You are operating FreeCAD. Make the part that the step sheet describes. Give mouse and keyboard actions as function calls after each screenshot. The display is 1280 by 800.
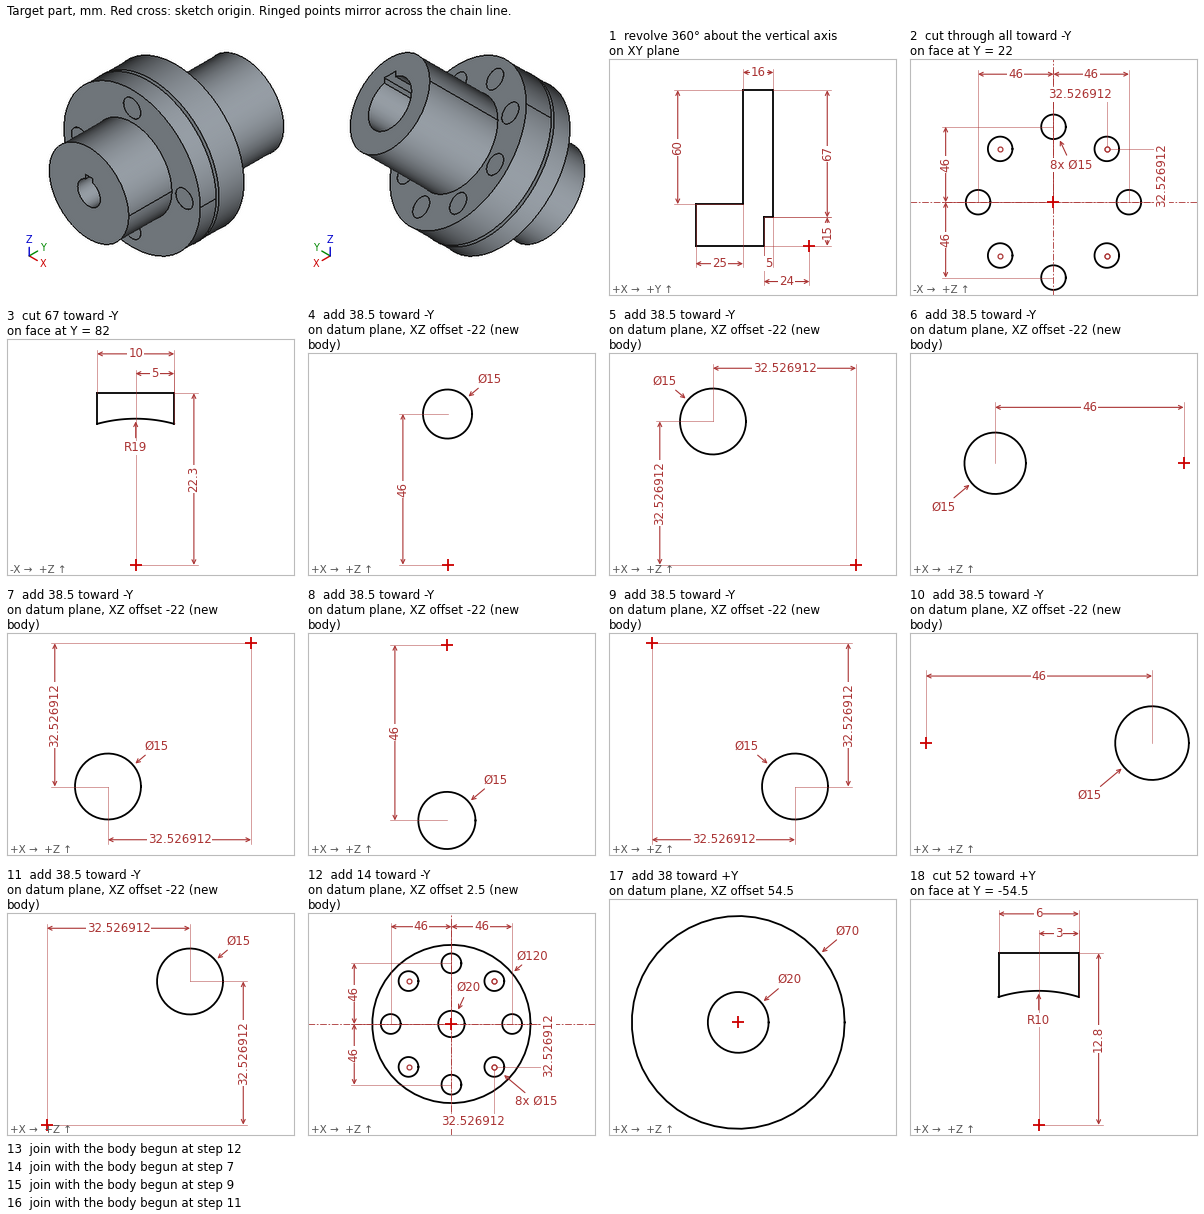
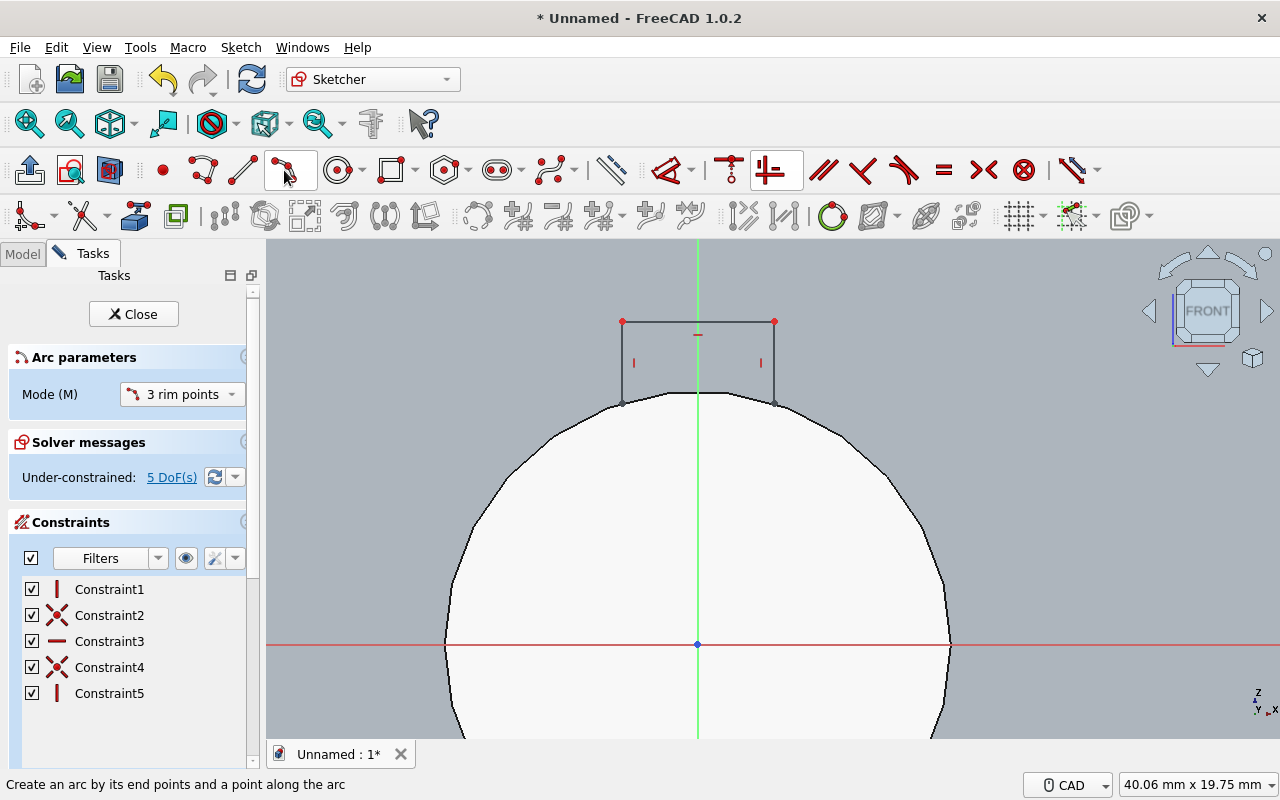
click(622, 404)
click(774, 404)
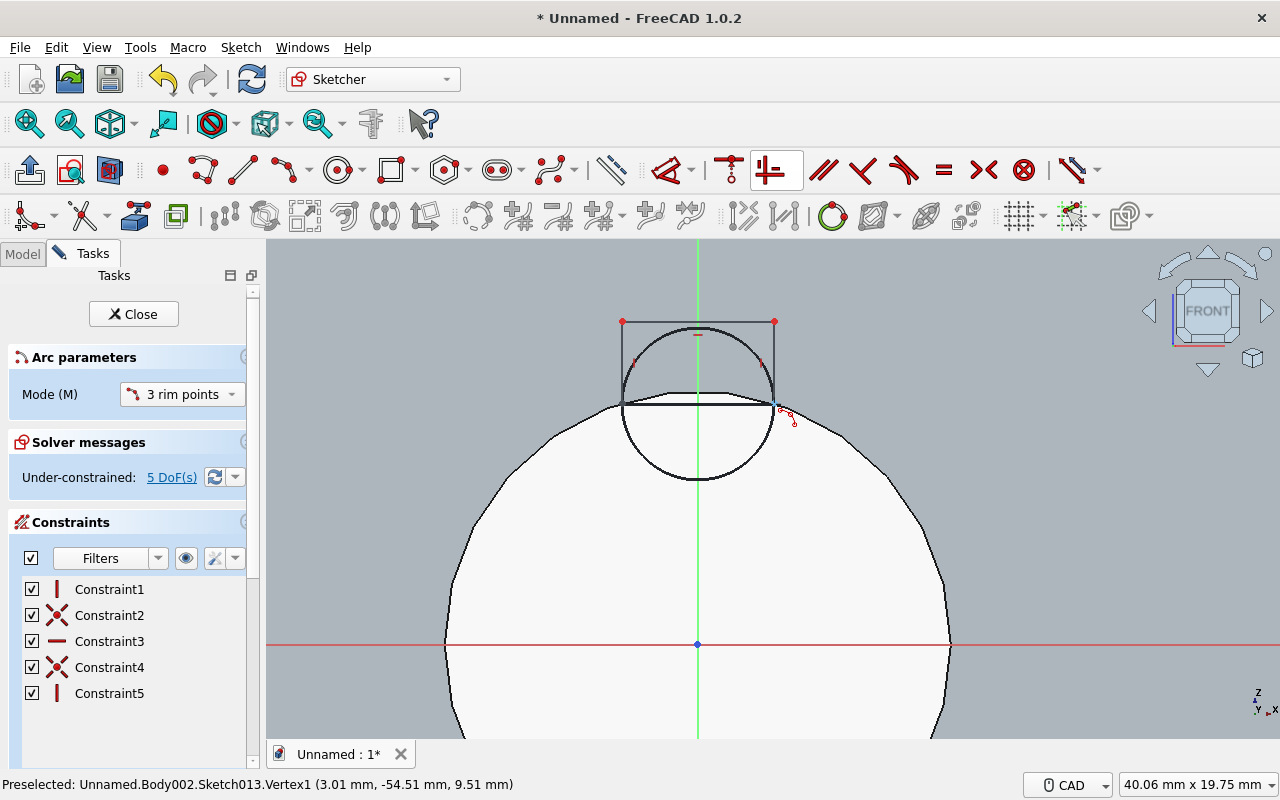
scroll(713, 392, up, 2)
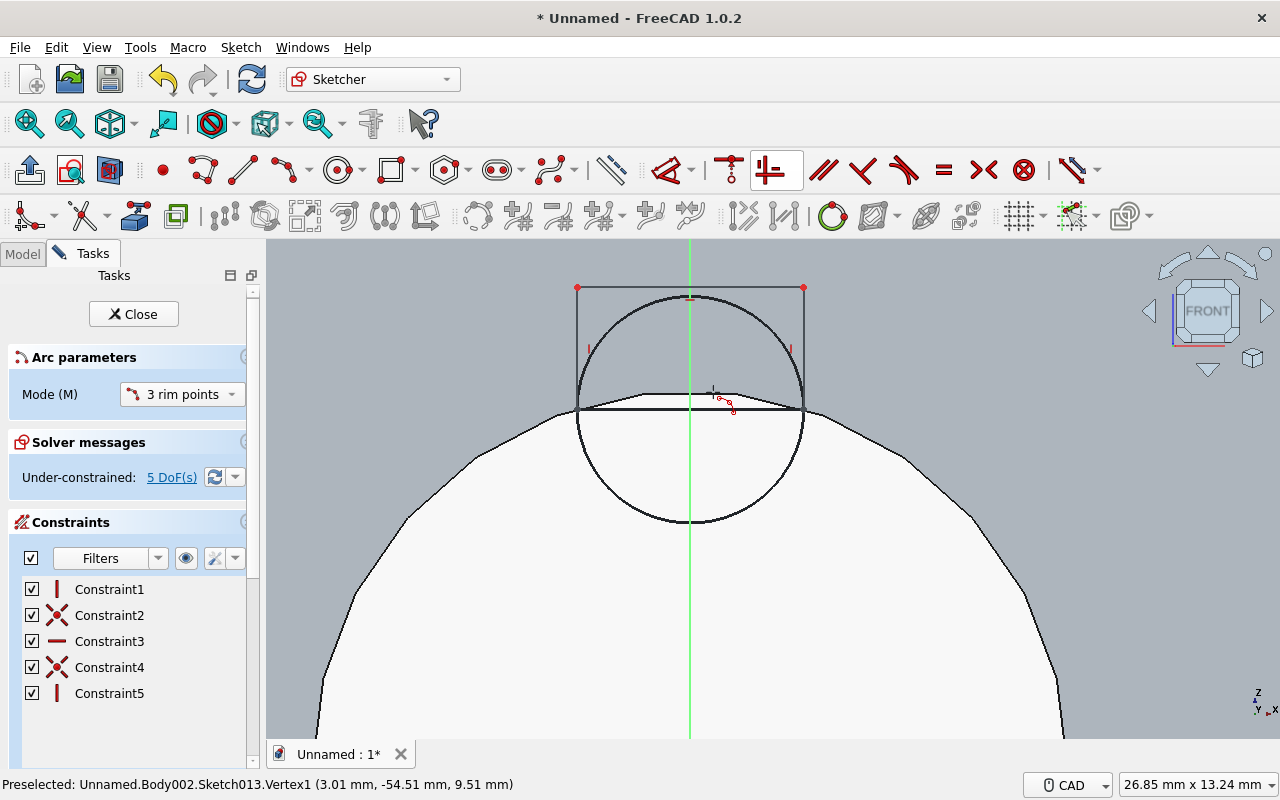
click(713, 392)
key(Escape)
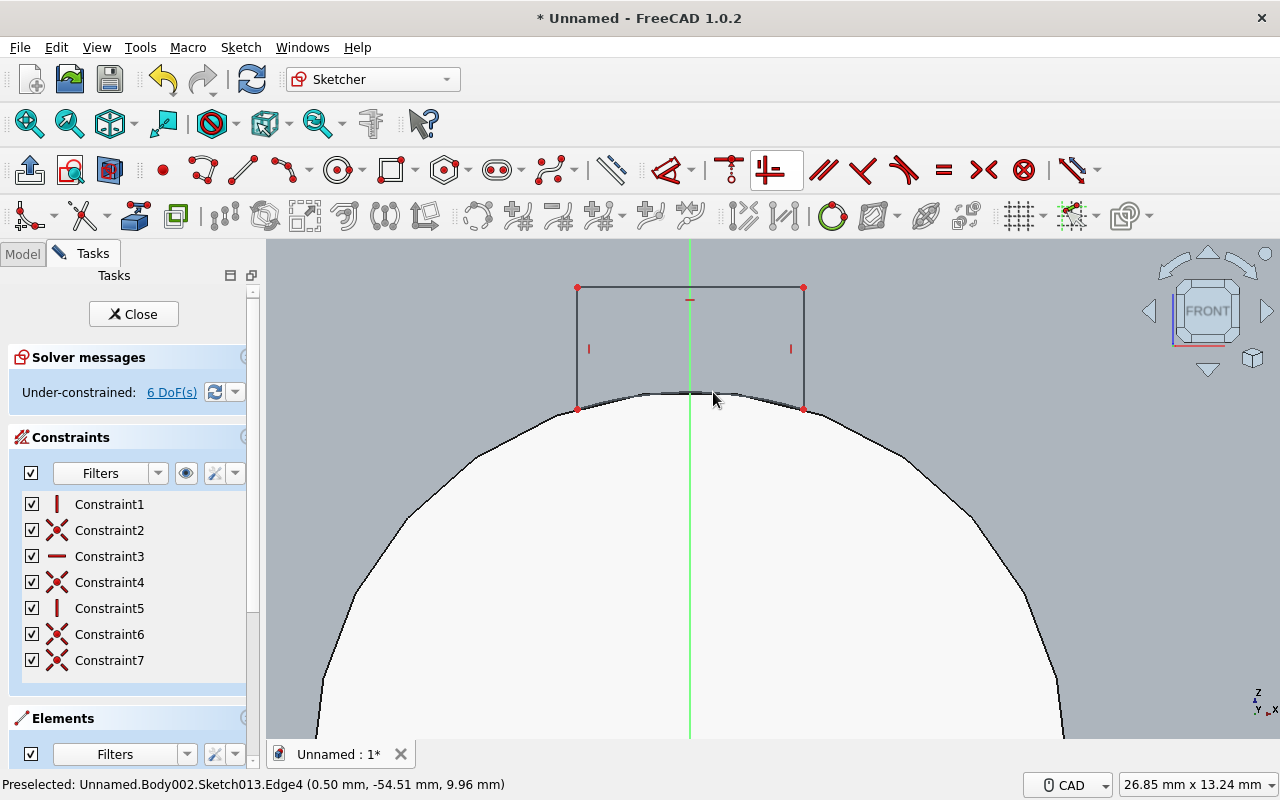
scroll(734, 411, down, 2)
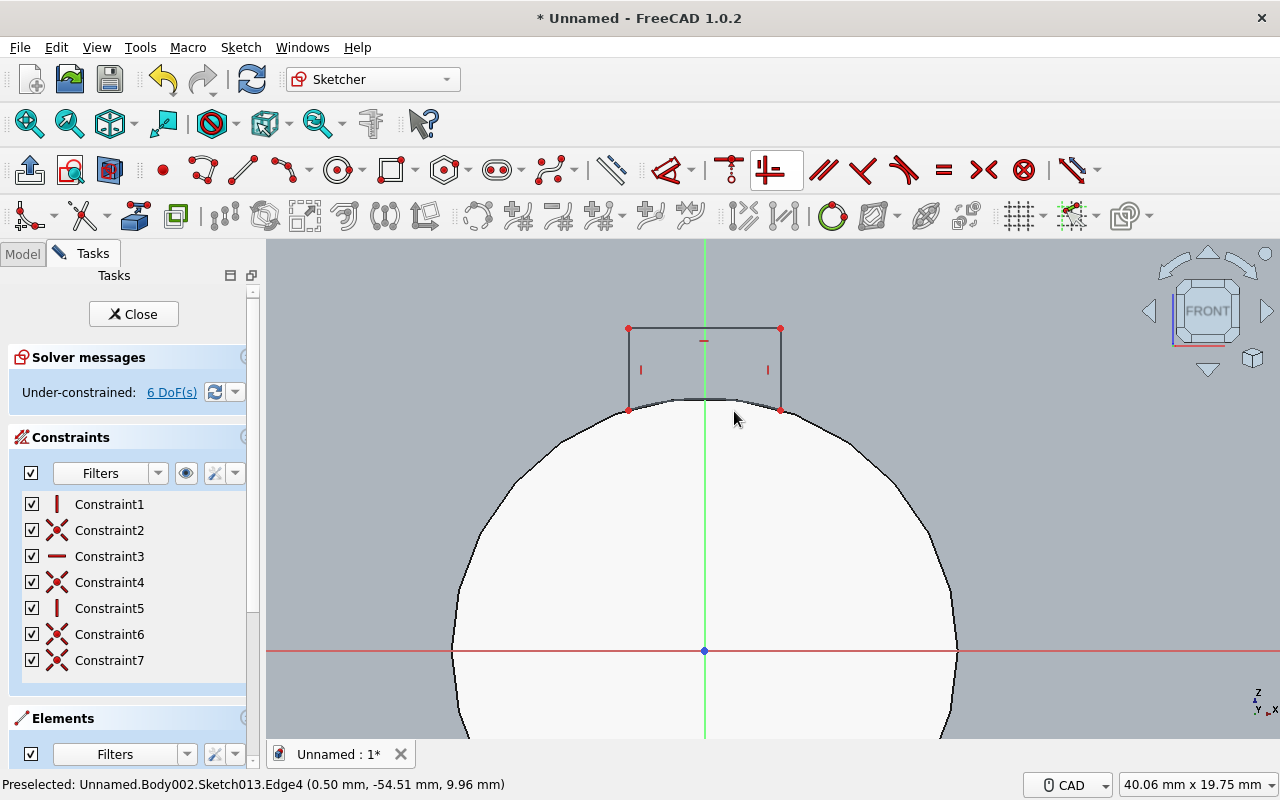
drag(695, 641, 715, 662)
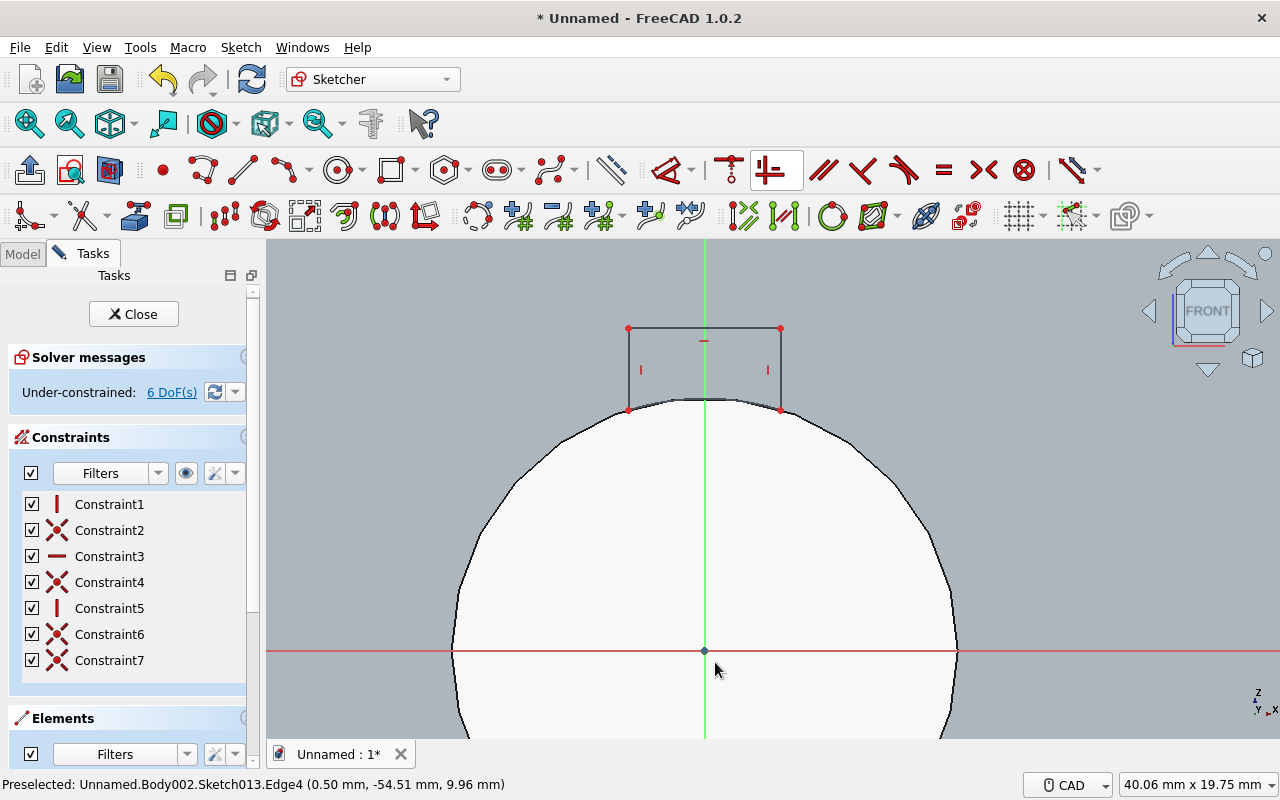
click(730, 170)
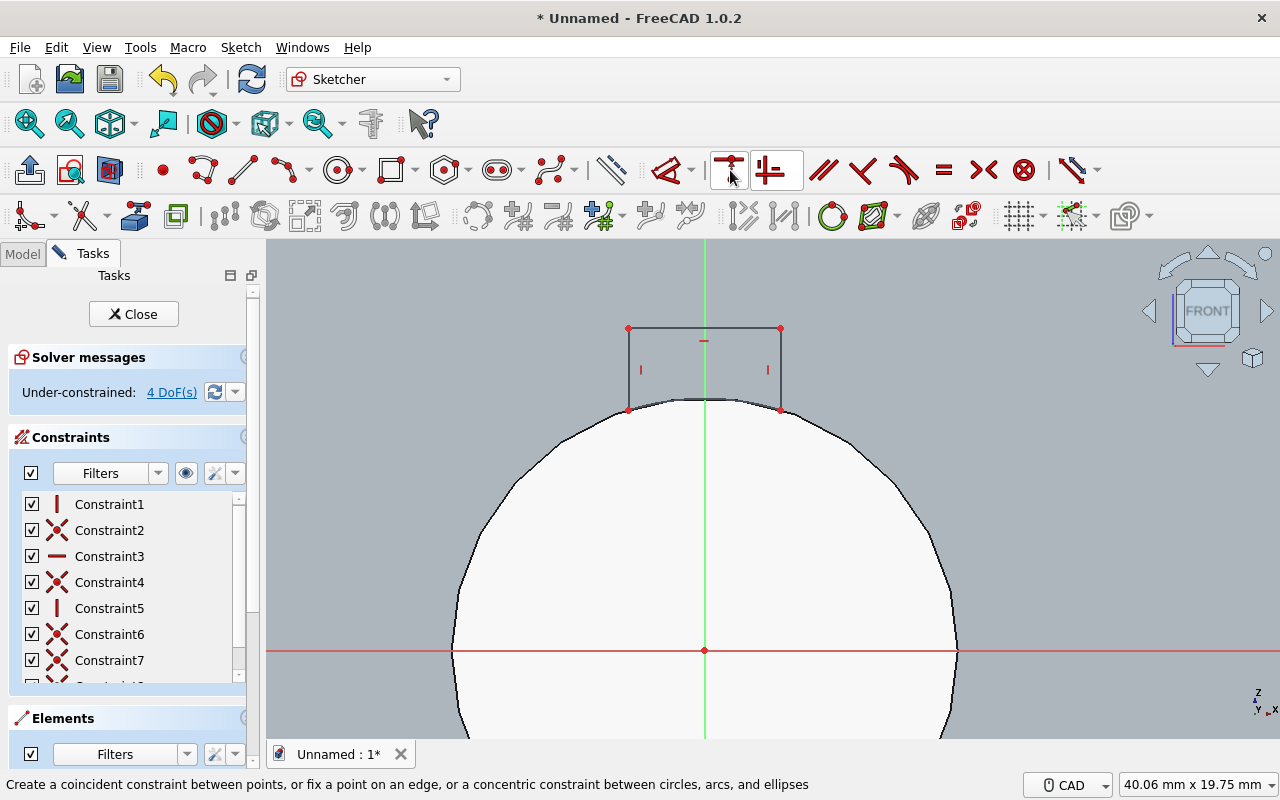
click(666, 170)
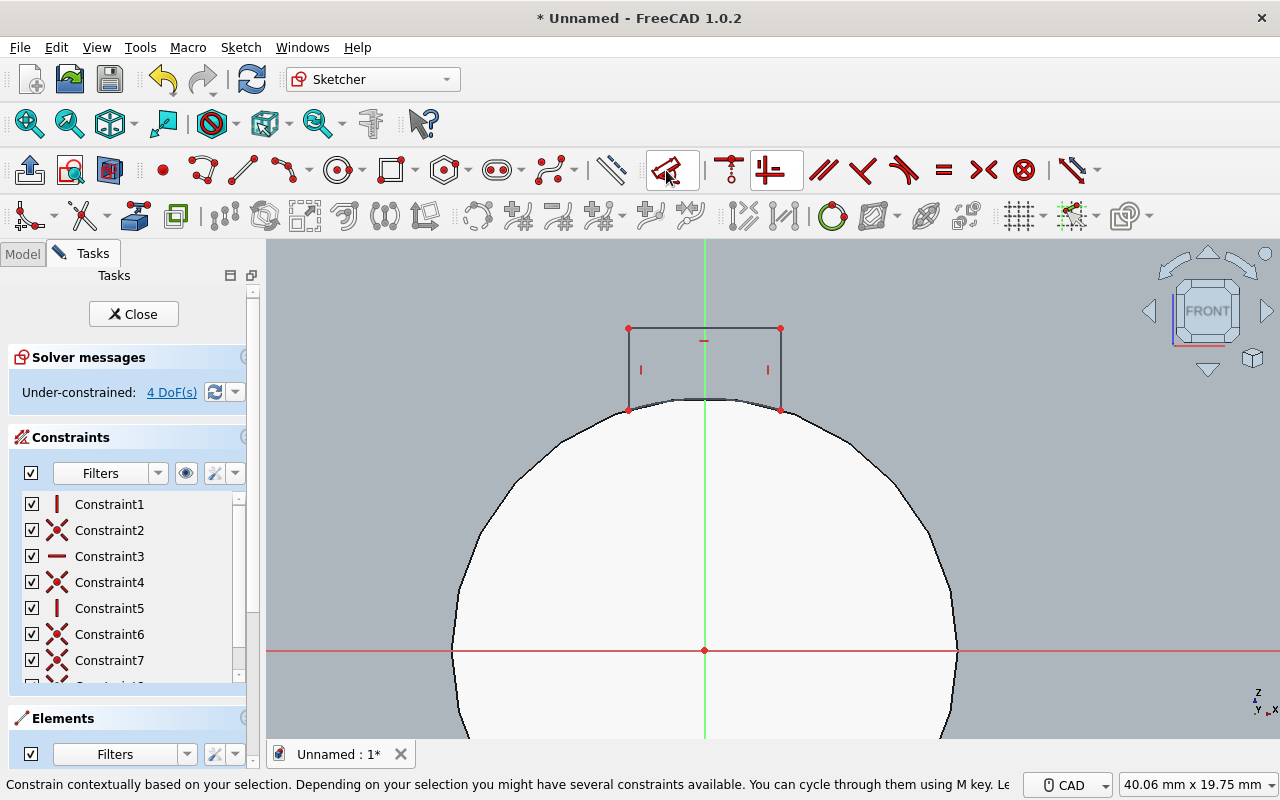
click(736, 401)
click(740, 369)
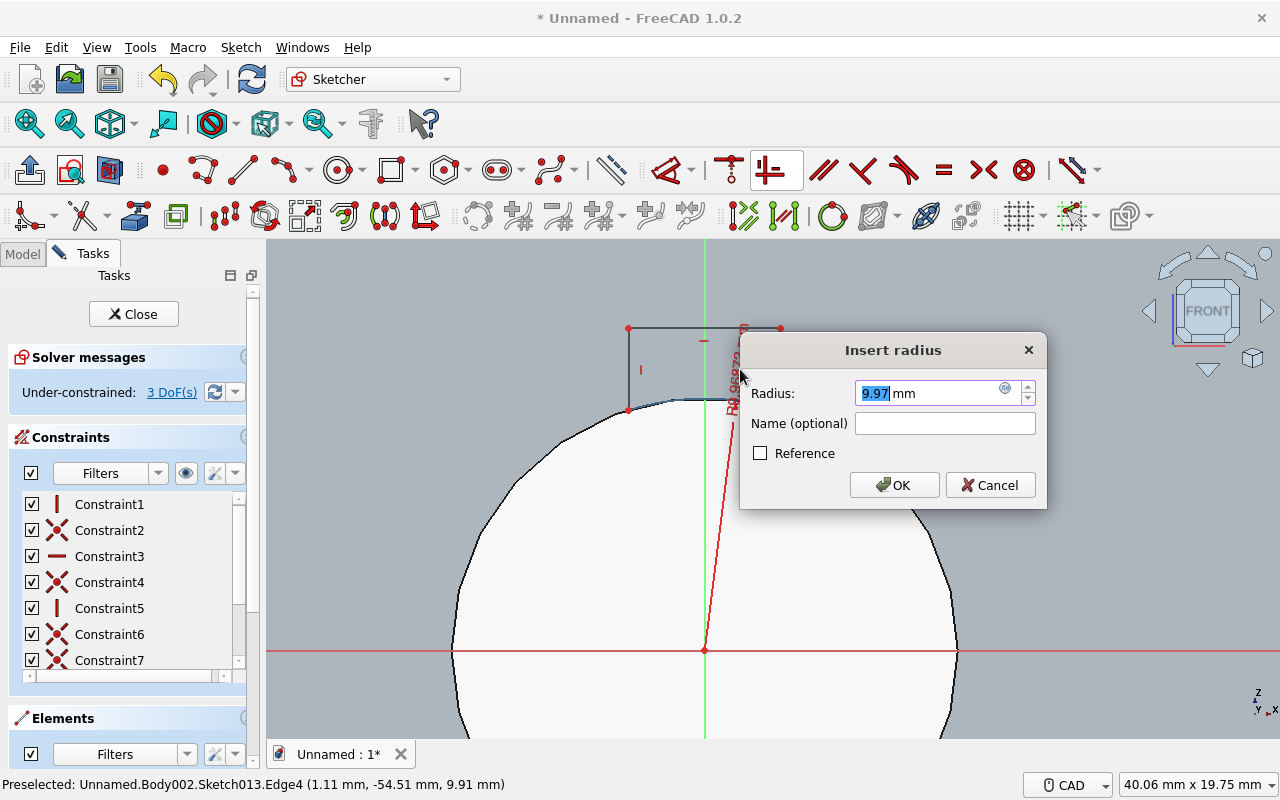
text(10)
key(Return)